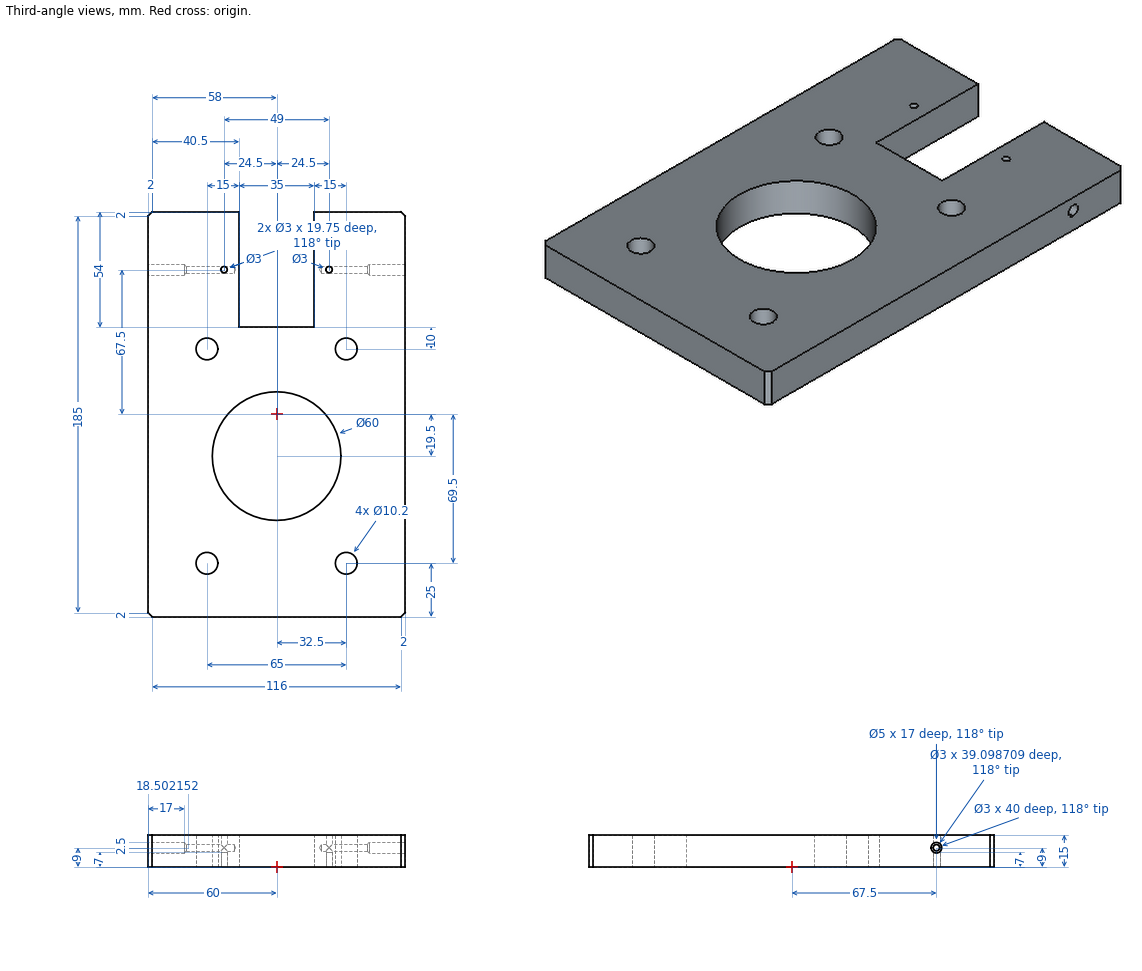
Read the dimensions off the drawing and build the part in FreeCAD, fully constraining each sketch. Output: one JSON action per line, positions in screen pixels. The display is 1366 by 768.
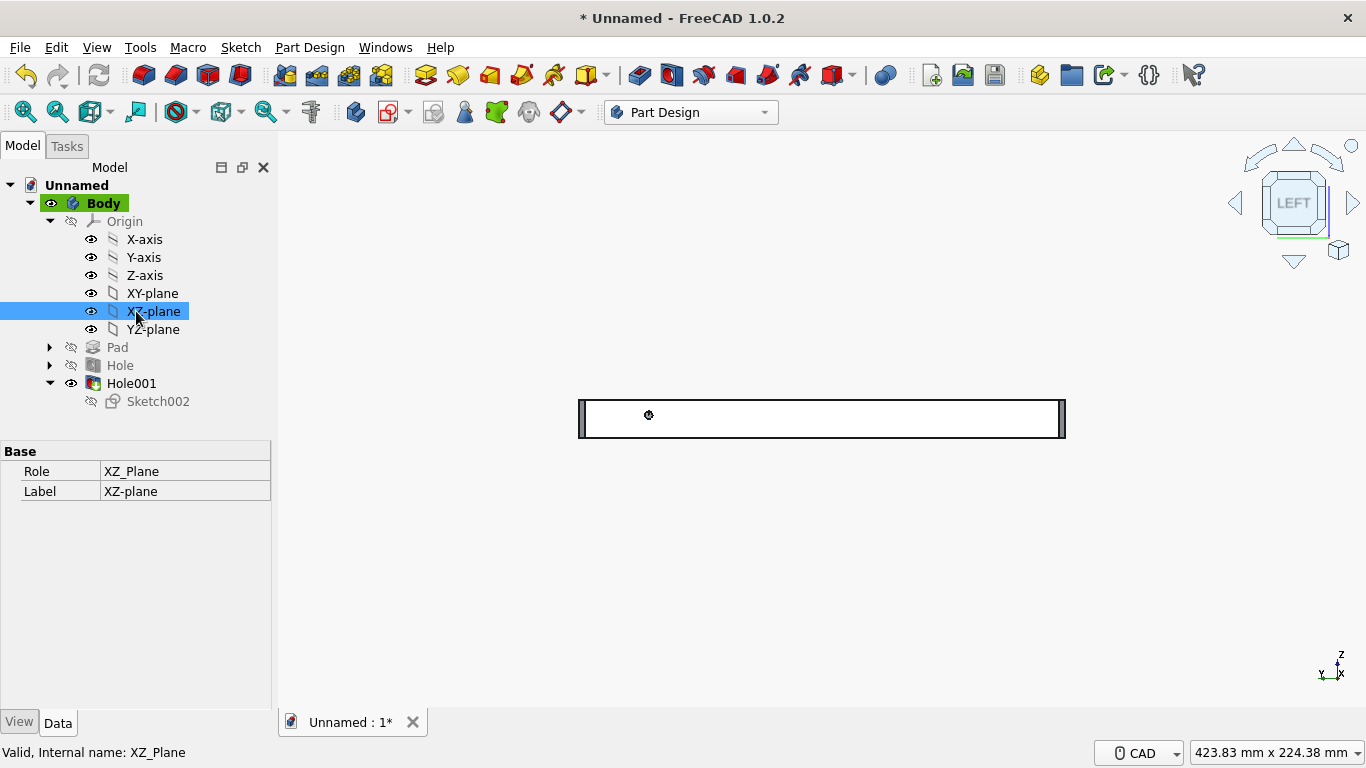
{"action": "left_click", "coordinate": [562, 112]}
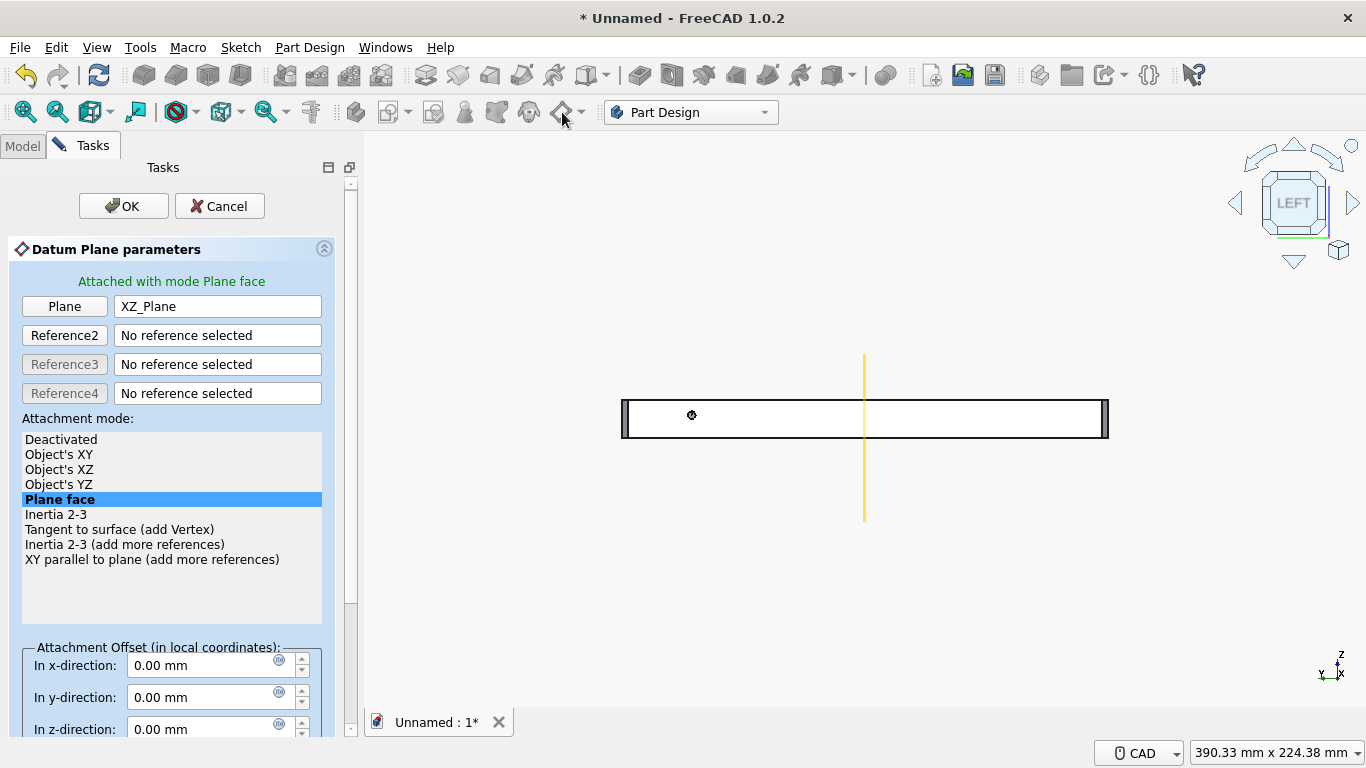
{"action": "scroll", "coordinate": [351, 456], "scroll_direction": "down", "scroll_amount": 2}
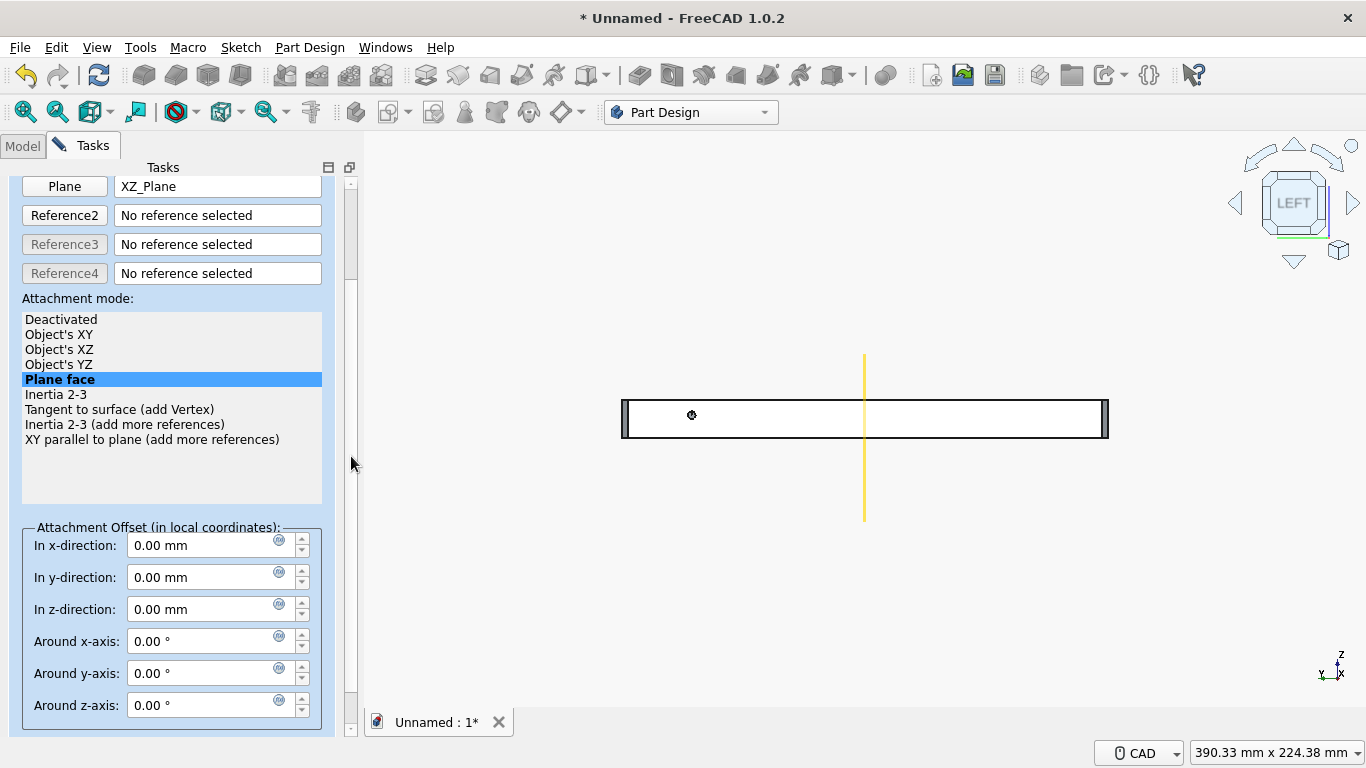
{"action": "triple_click", "coordinate": [210, 609]}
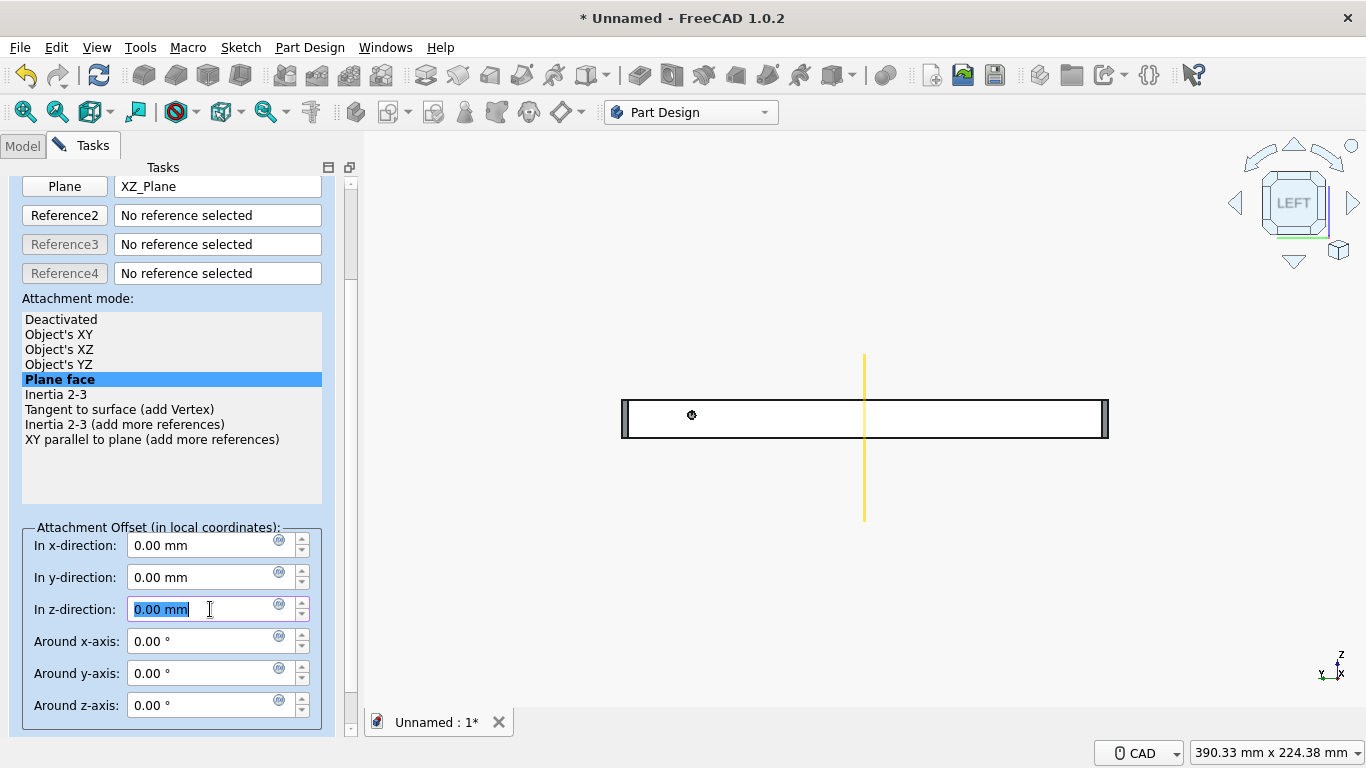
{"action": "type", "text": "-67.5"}
{"action": "key", "text": "Tab"}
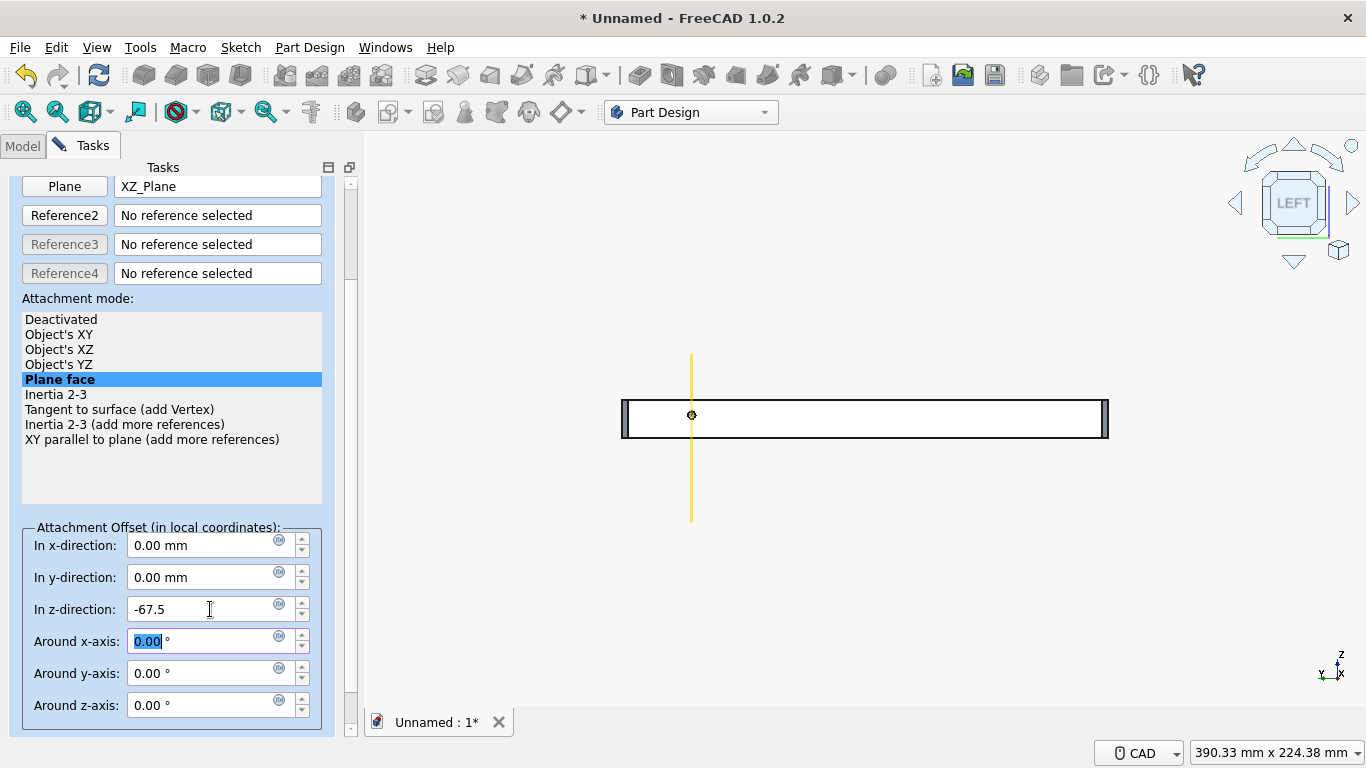
{"action": "scroll", "coordinate": [351, 456], "scroll_direction": "up", "scroll_amount": 3}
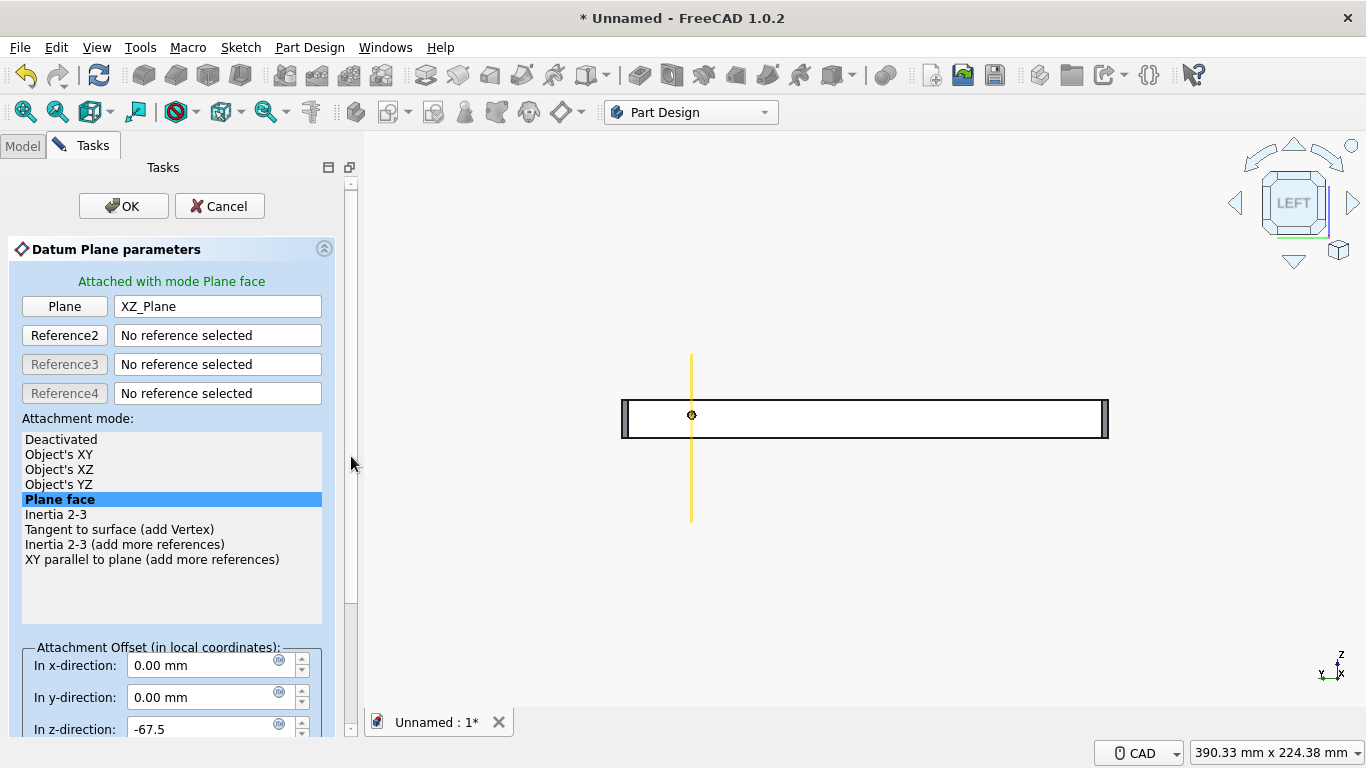
{"action": "left_click", "coordinate": [124, 206]}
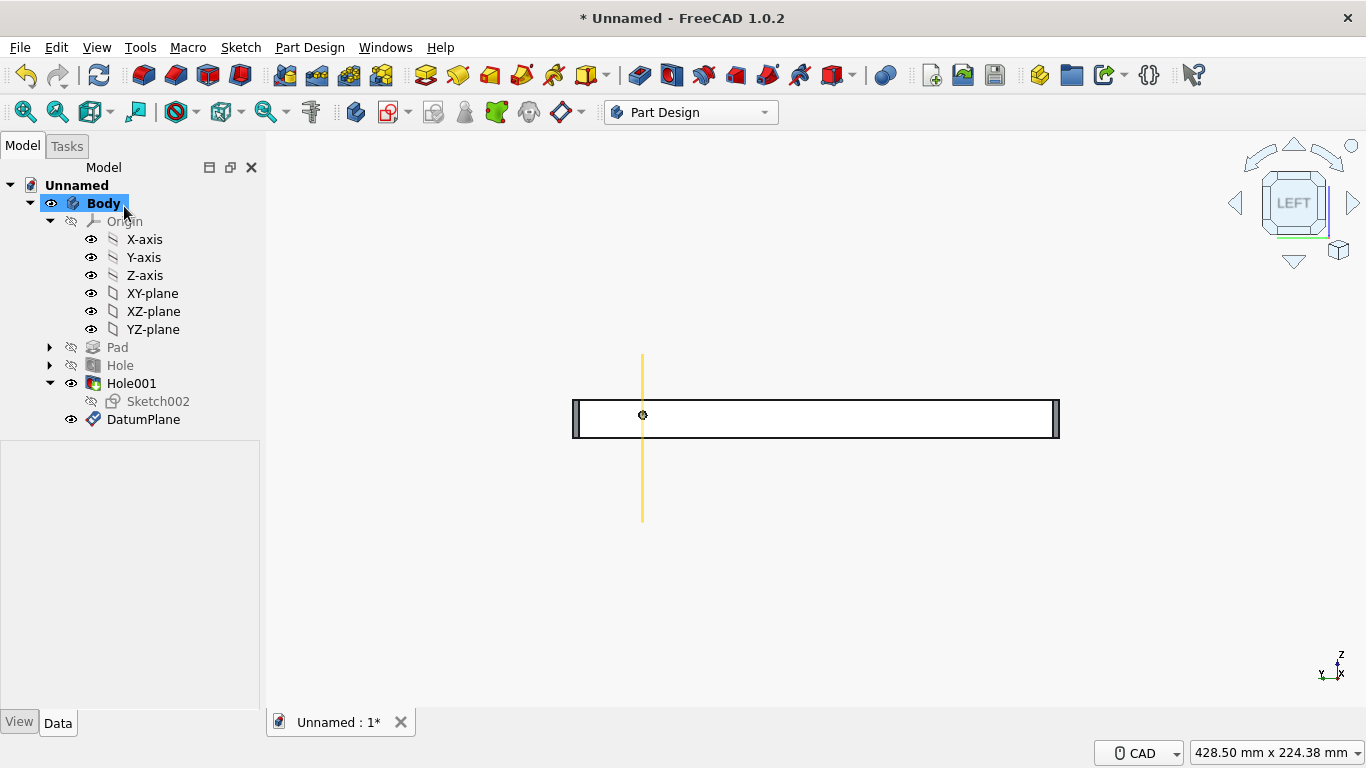
{"action": "left_click", "coordinate": [116, 419]}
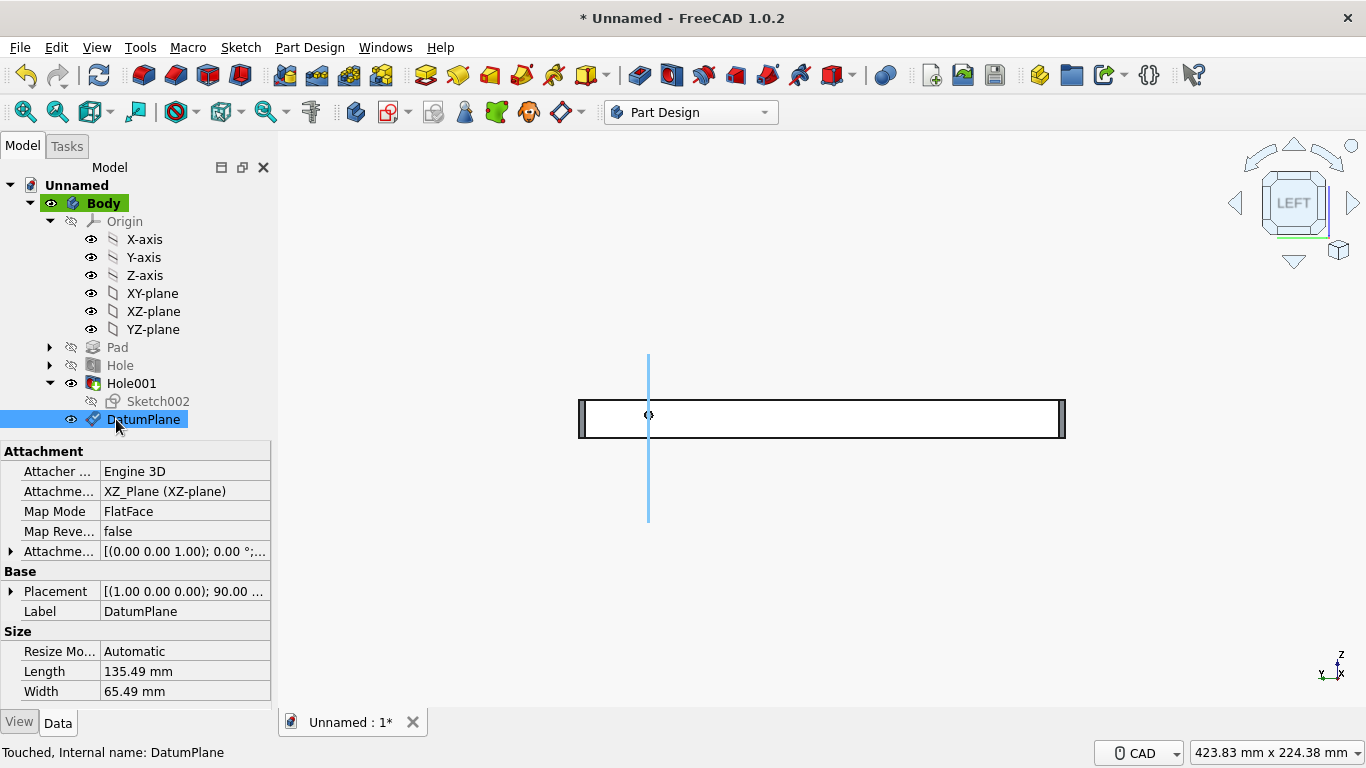
{"action": "left_click", "coordinate": [388, 112]}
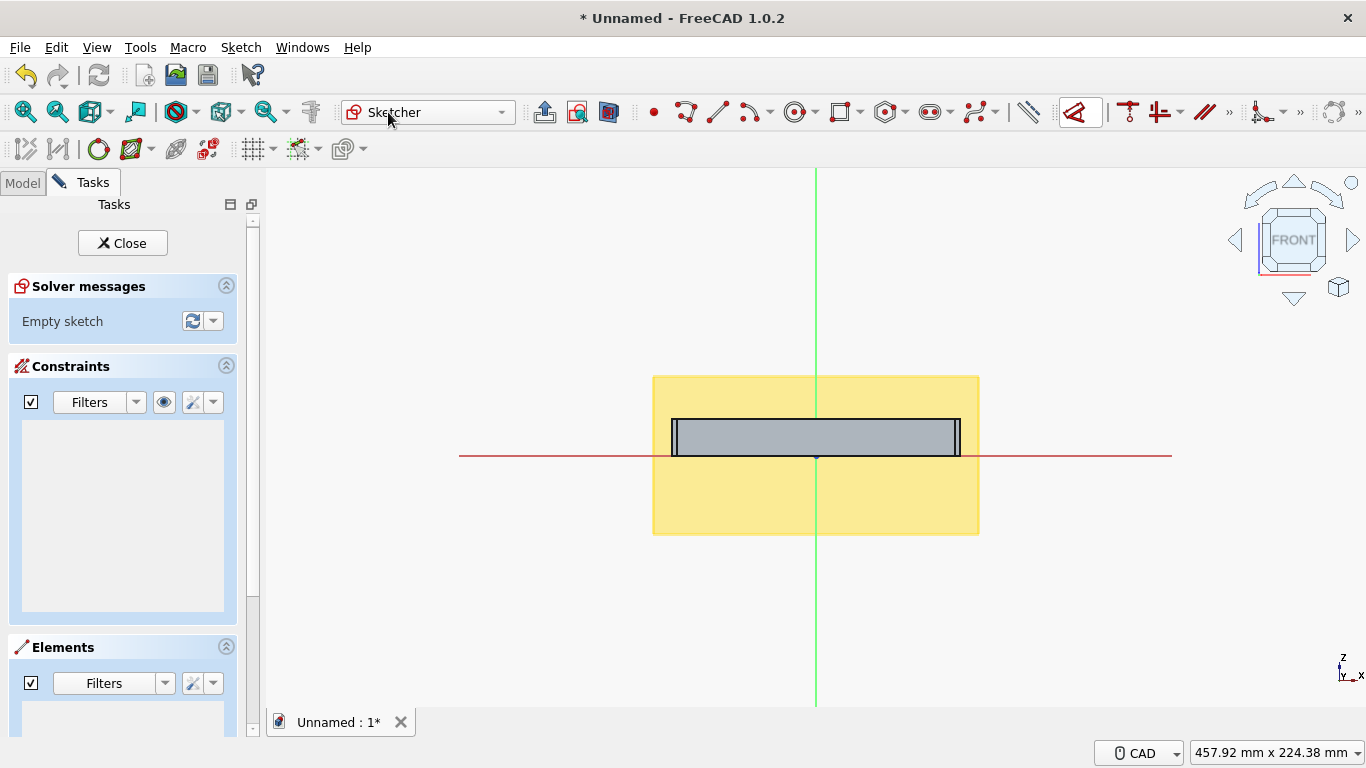
{"action": "key", "text": "q s"}